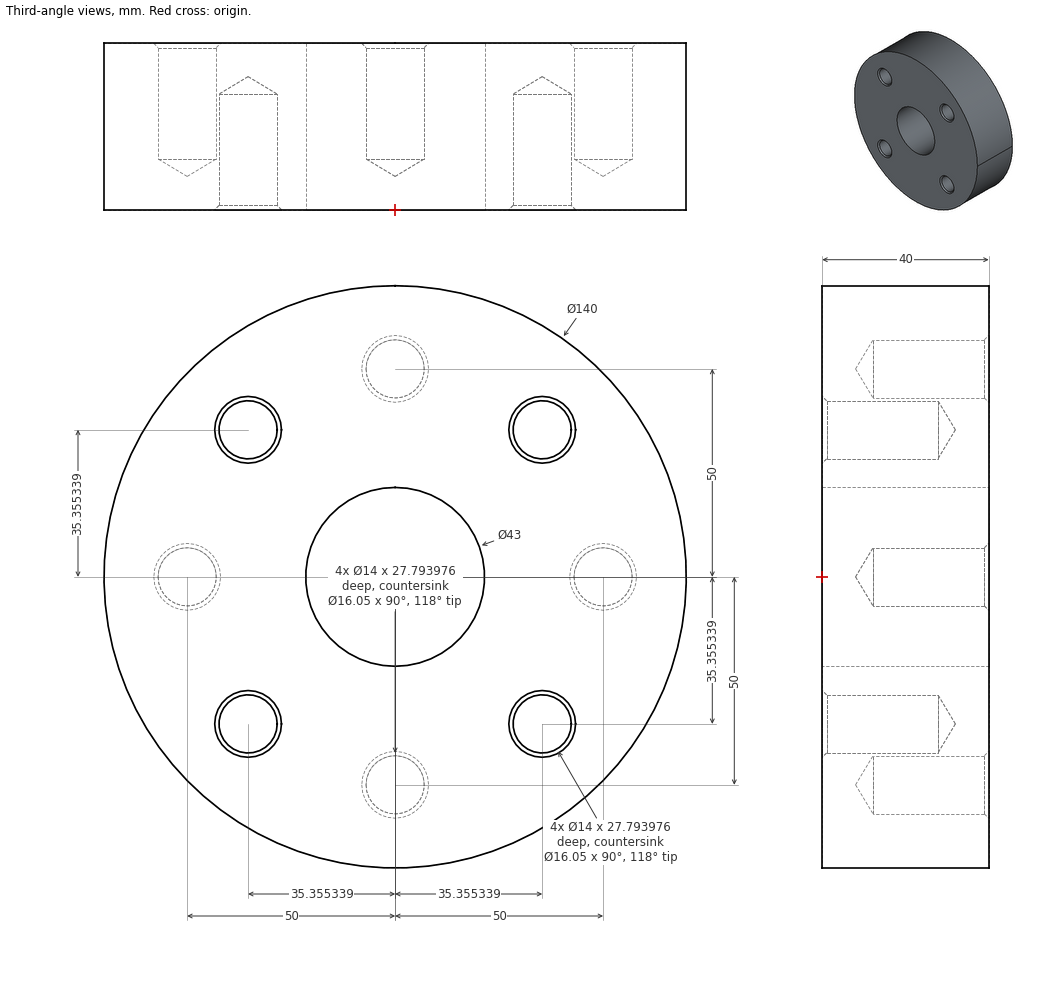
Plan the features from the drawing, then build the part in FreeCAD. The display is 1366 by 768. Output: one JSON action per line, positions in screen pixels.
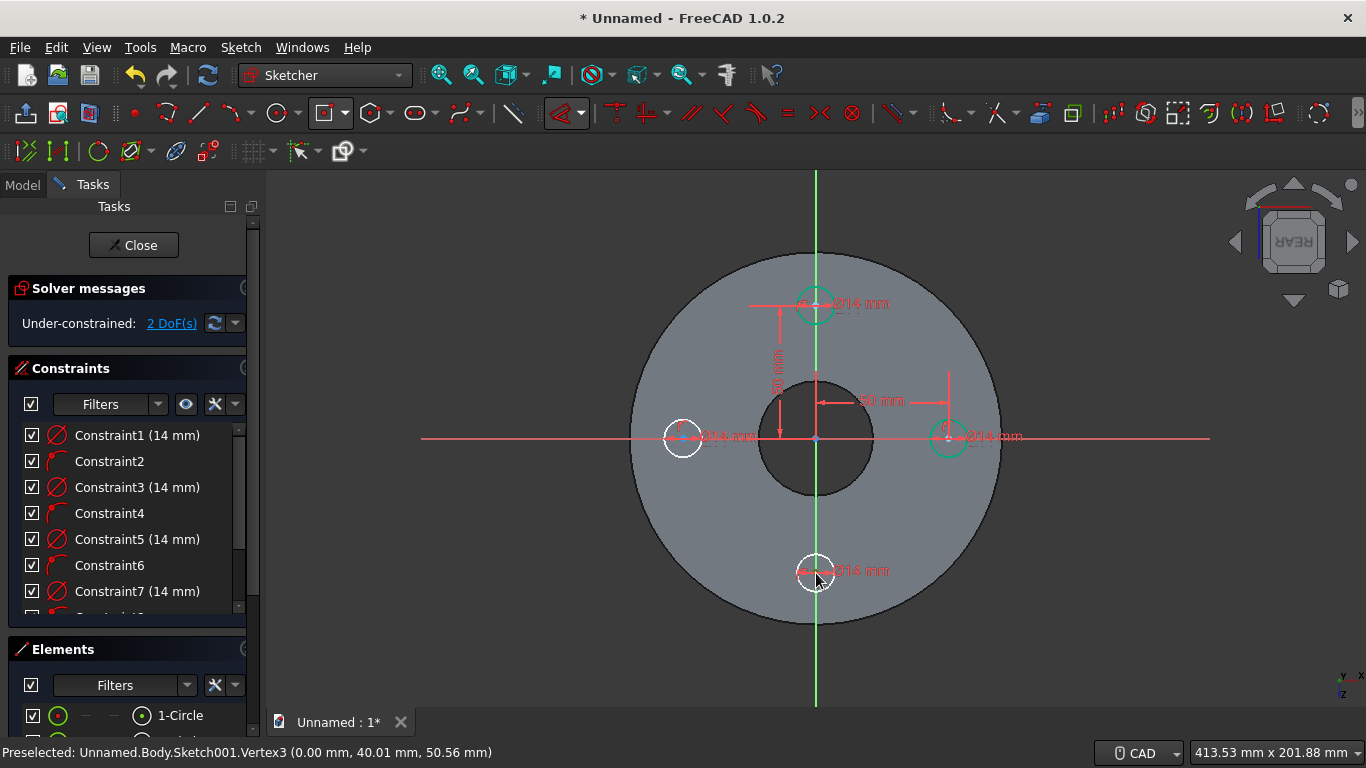
{"action": "key", "text": "i"}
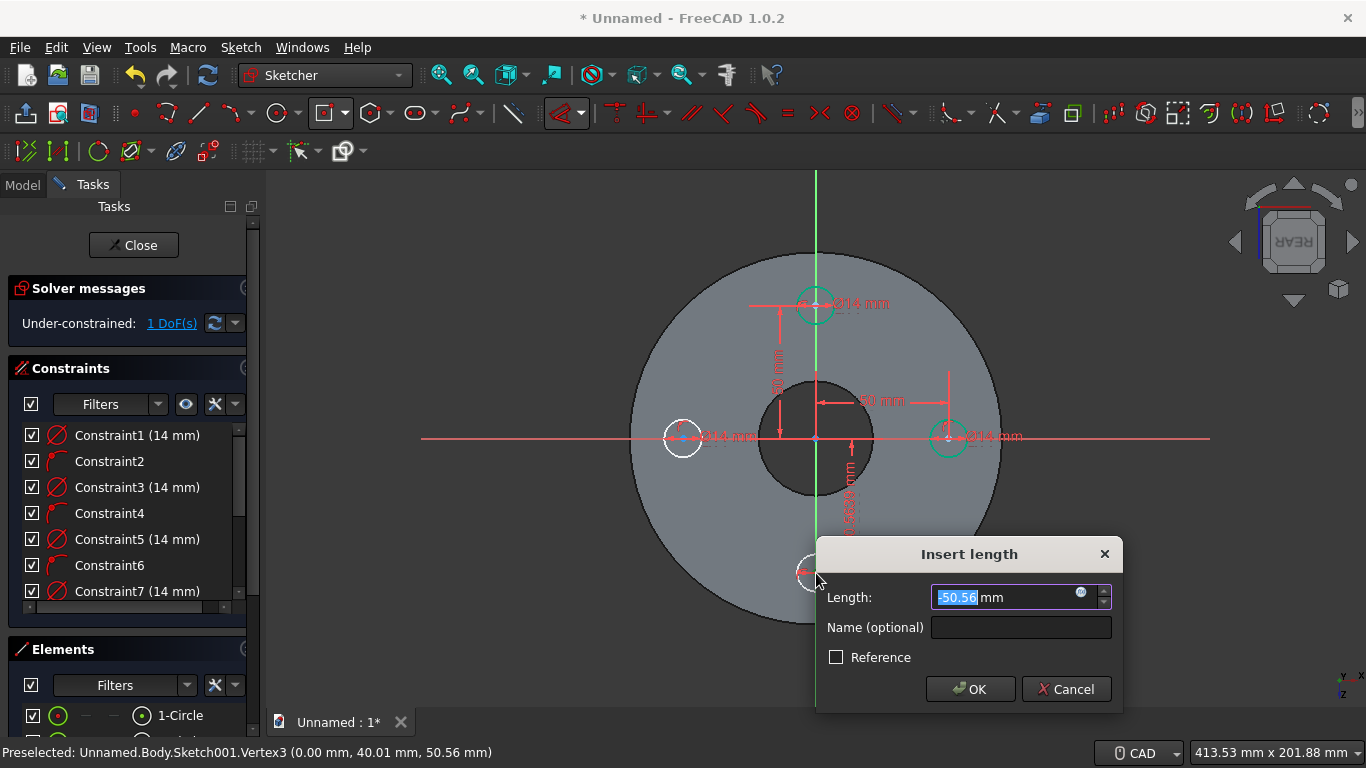
{"action": "type", "text": "-50"}
{"action": "key", "text": "Return"}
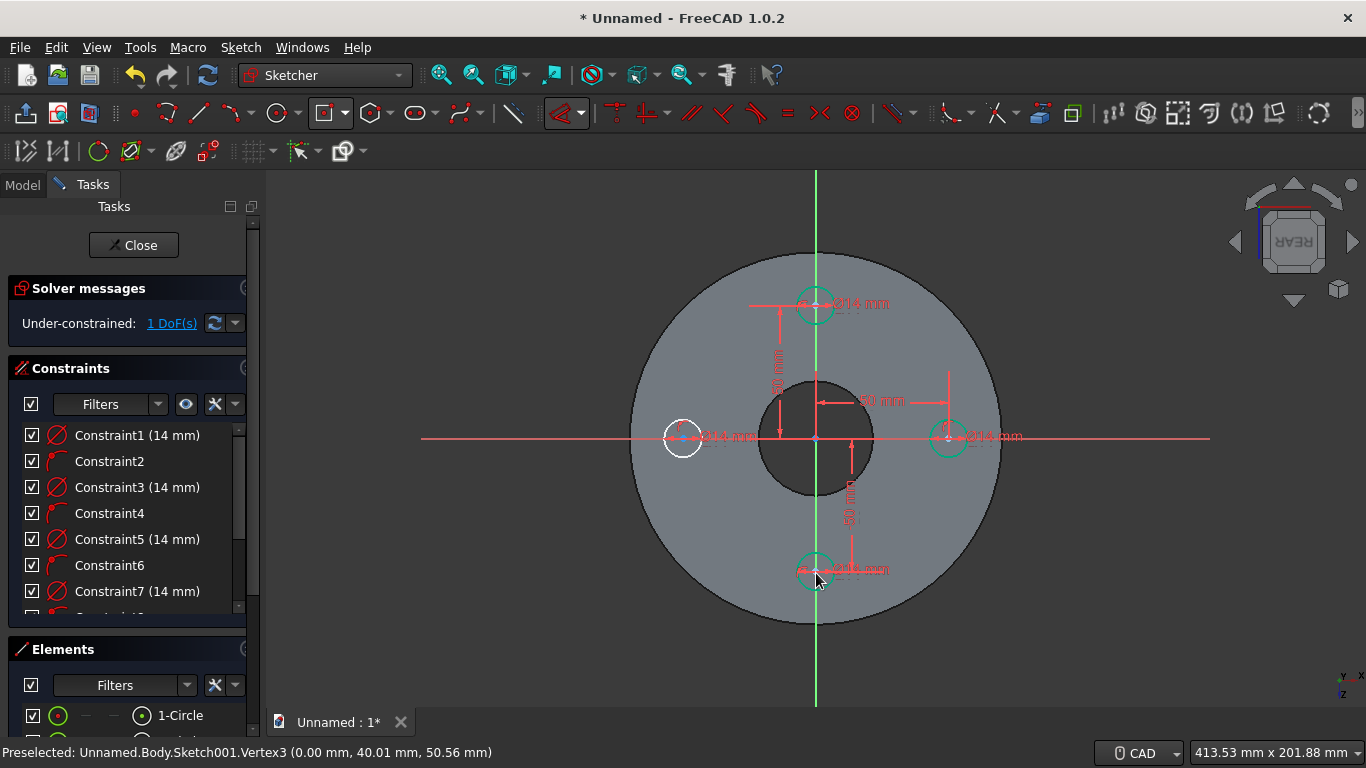
{"action": "left_click", "coordinate": [683, 439]}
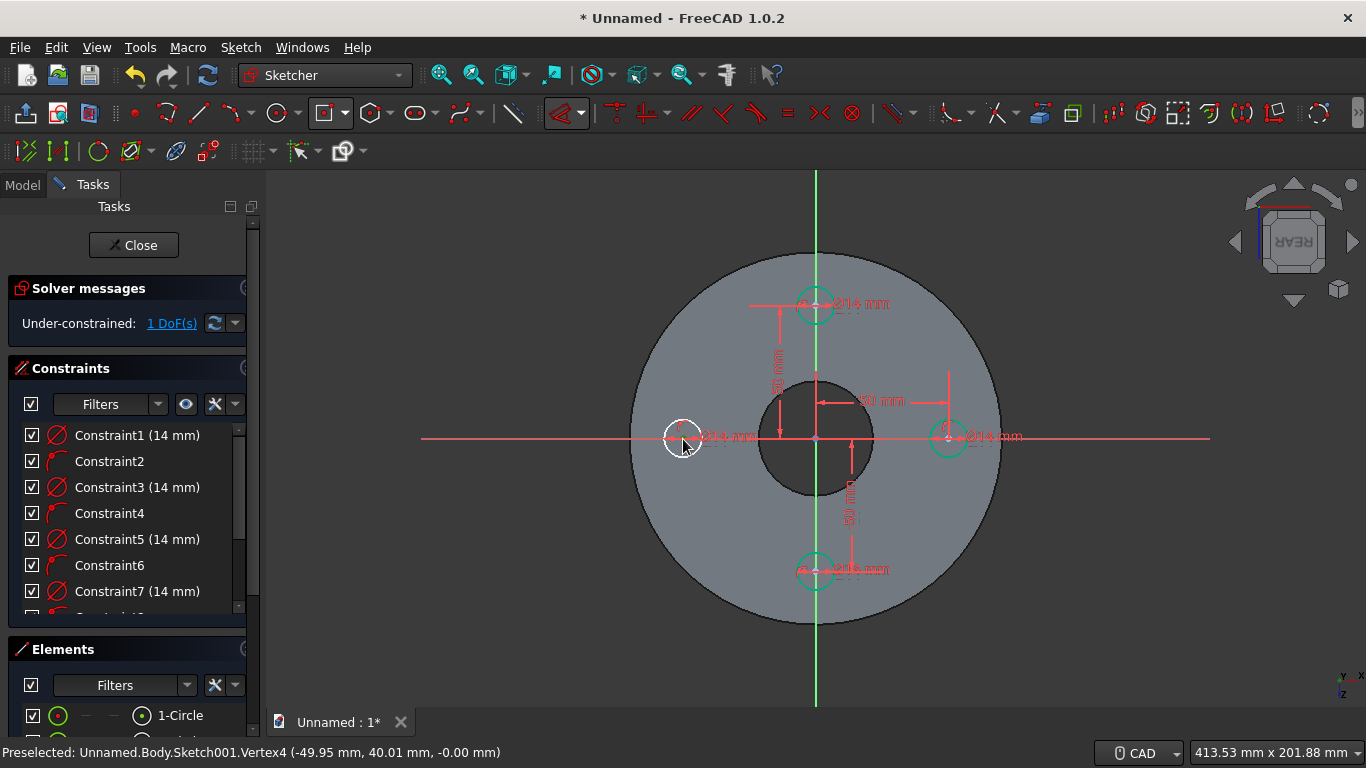
{"action": "key", "text": "l"}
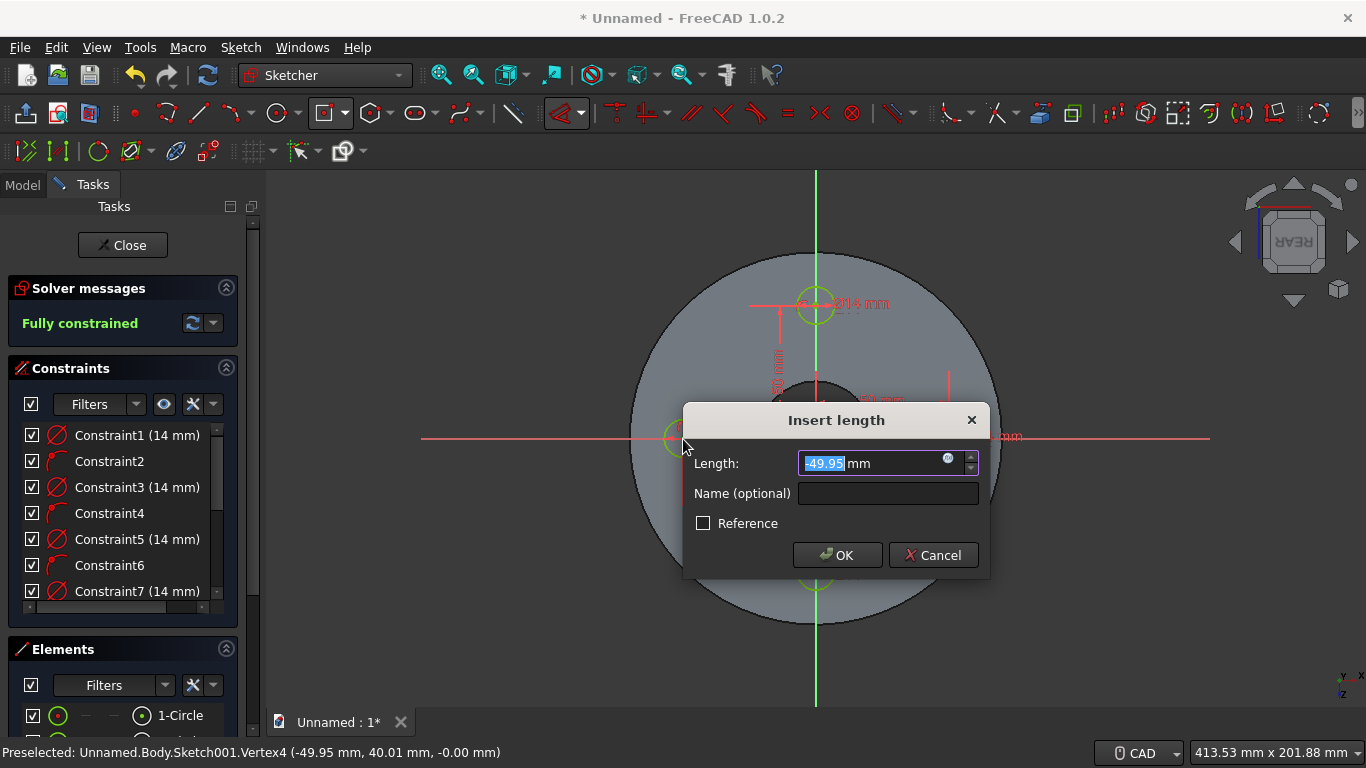
{"action": "type", "text": "-50"}
{"action": "key", "text": "Return"}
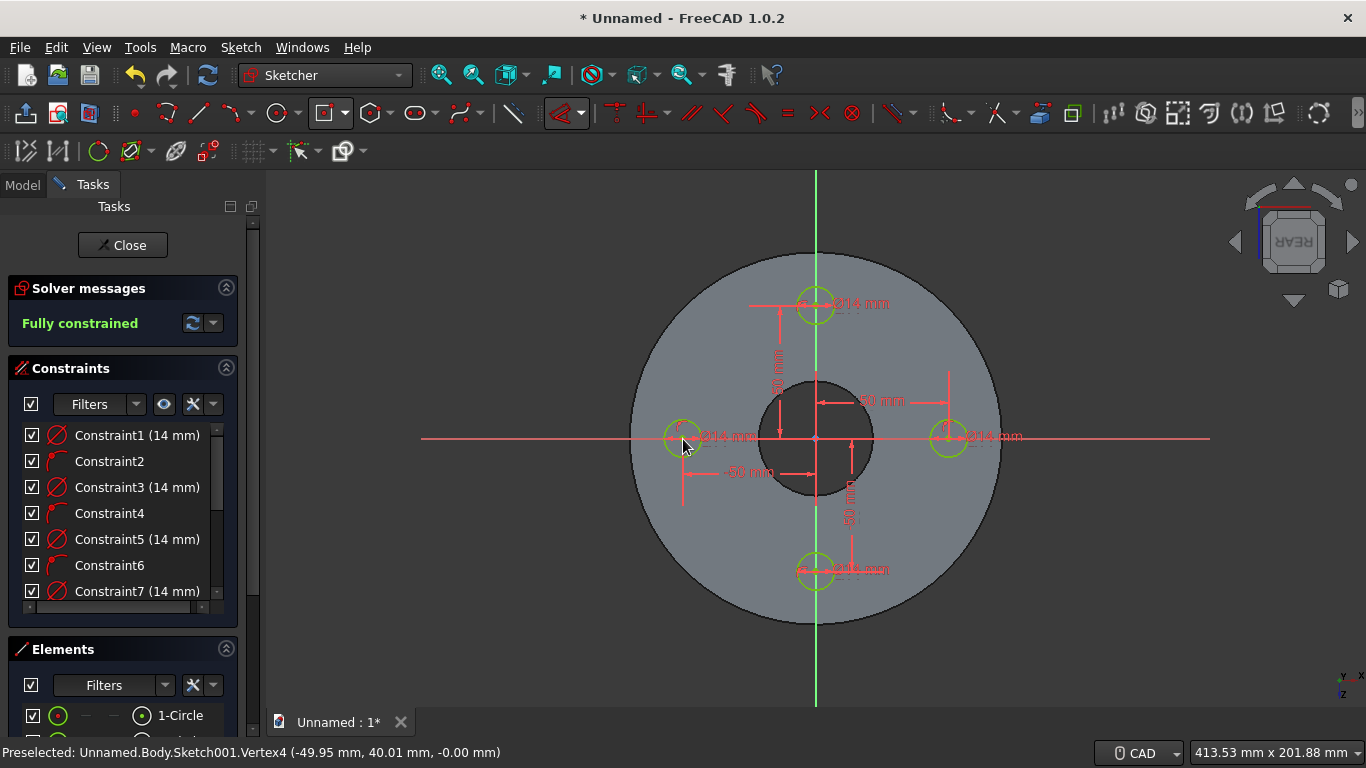
{"action": "left_click", "coordinate": [123, 245]}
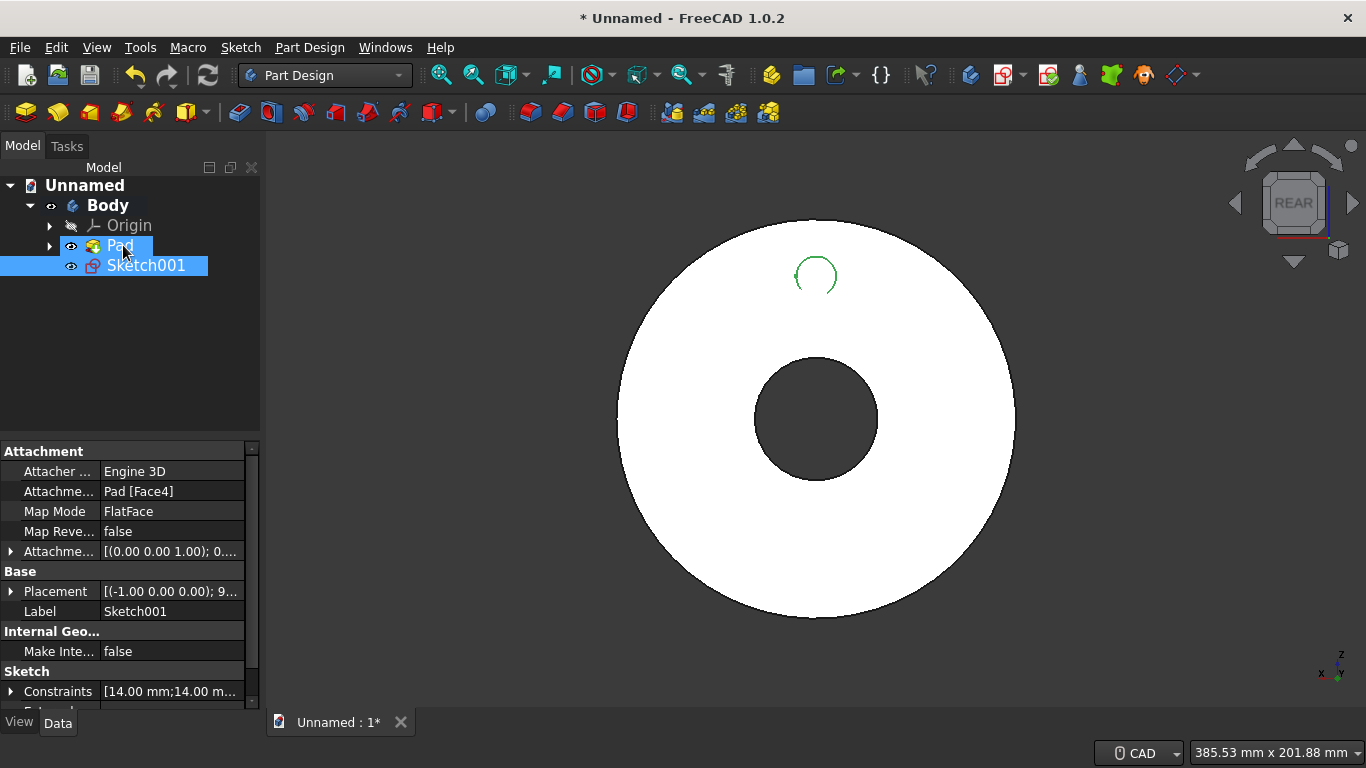
{"action": "left_click", "coordinate": [272, 112]}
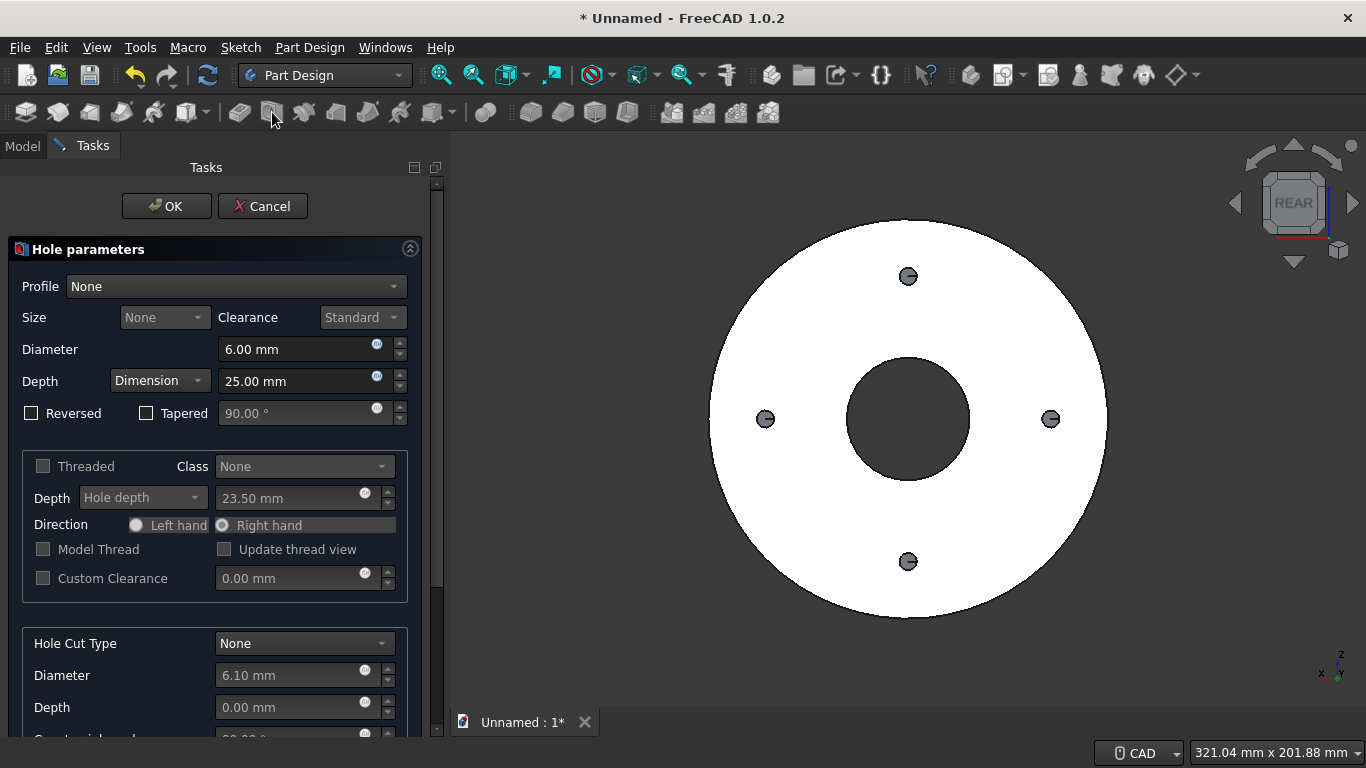
{"action": "triple_click", "coordinate": [305, 349]}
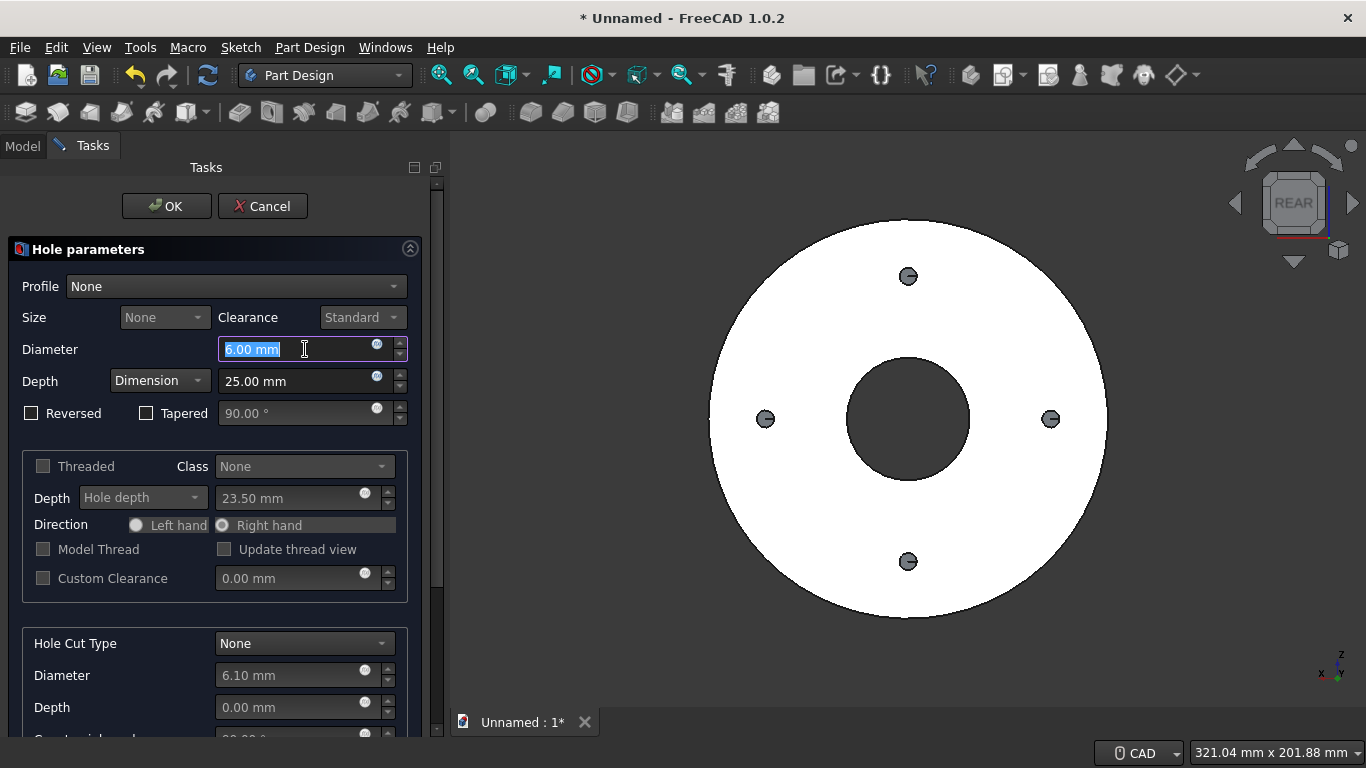
{"action": "type", "text": "14"}
{"action": "key", "text": "Tab"}